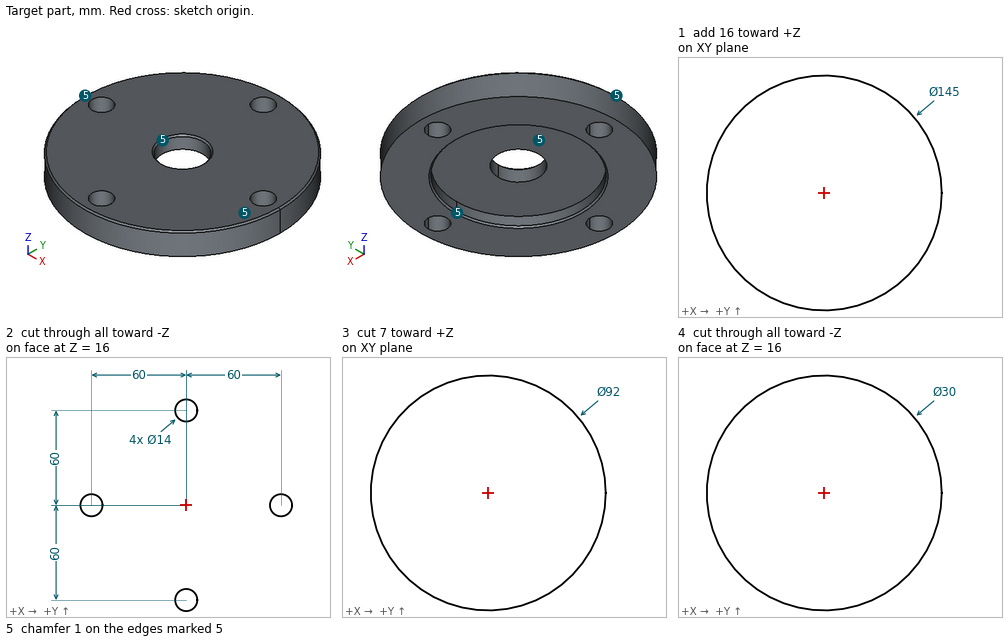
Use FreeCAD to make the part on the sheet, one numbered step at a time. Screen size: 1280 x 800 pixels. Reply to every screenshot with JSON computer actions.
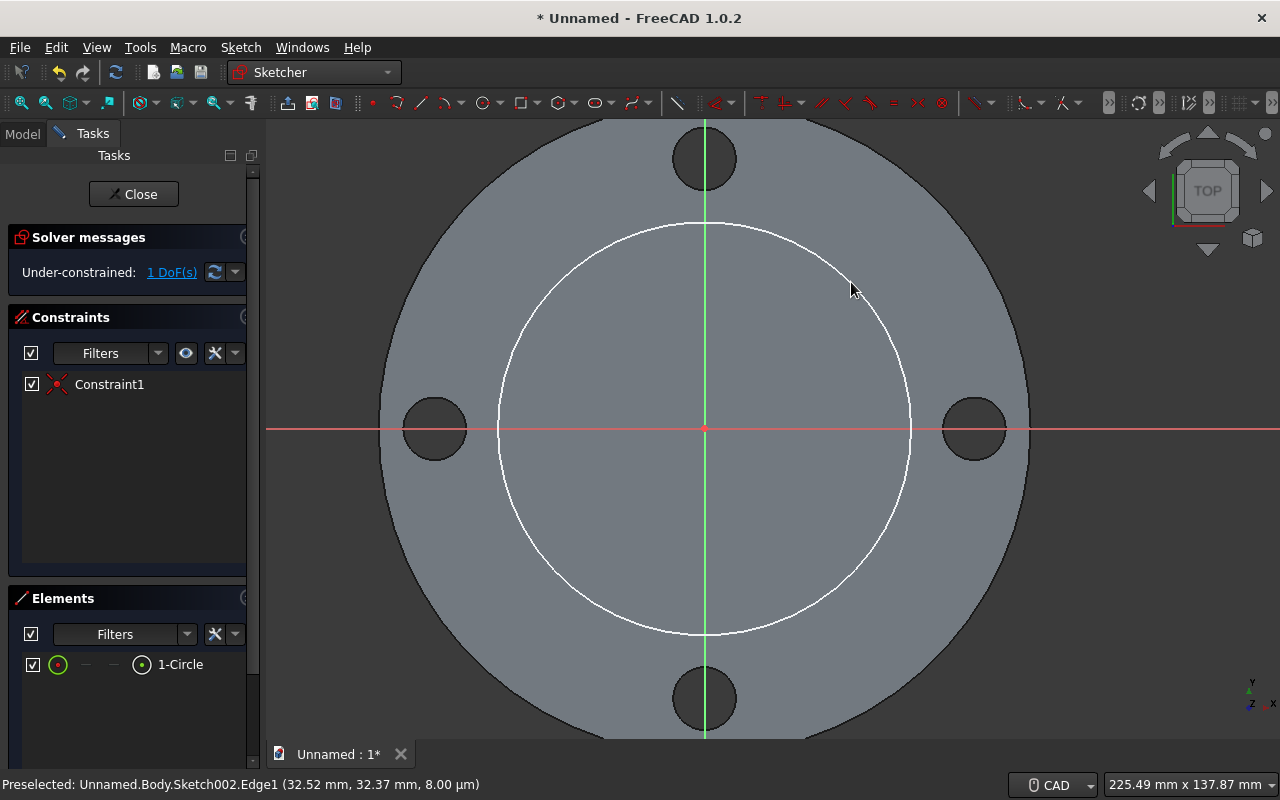
{"action": "left_click", "coordinate": [716, 104]}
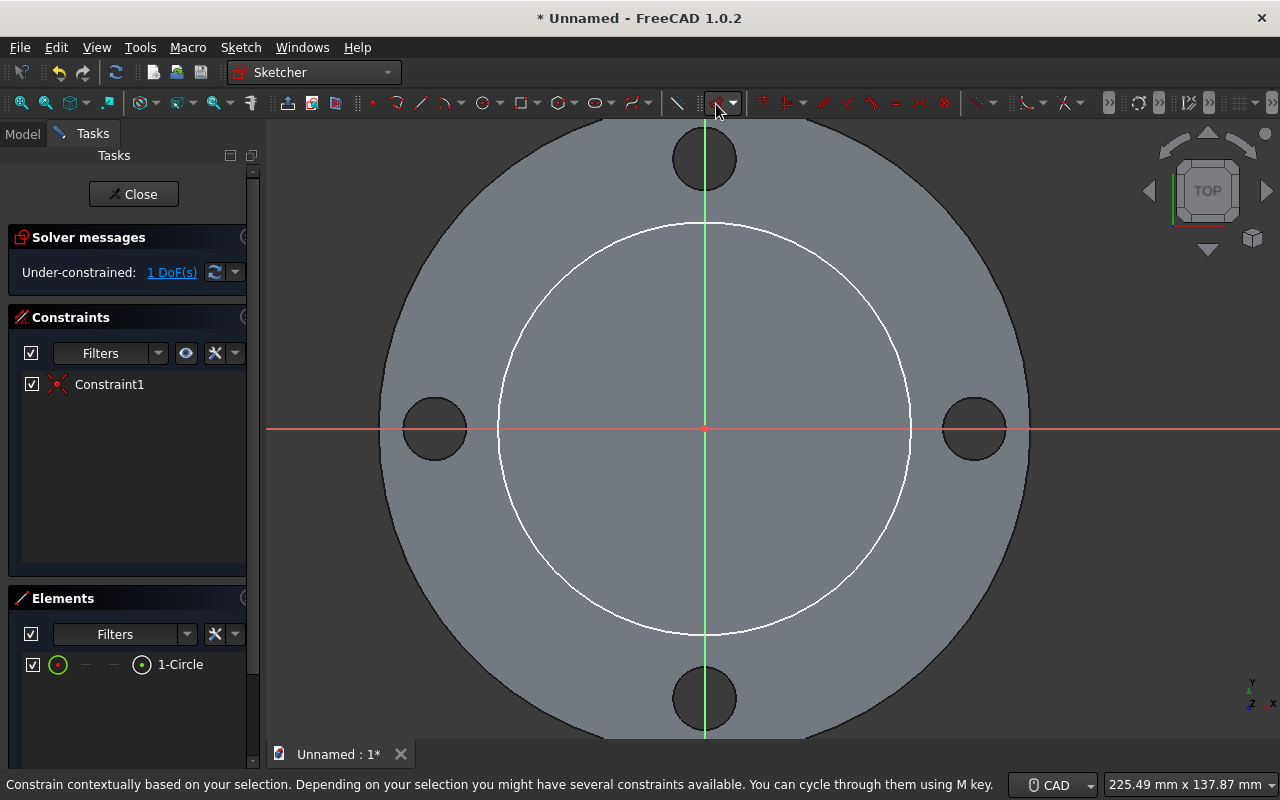
{"action": "left_click", "coordinate": [850, 282]}
{"action": "left_click", "coordinate": [873, 259]}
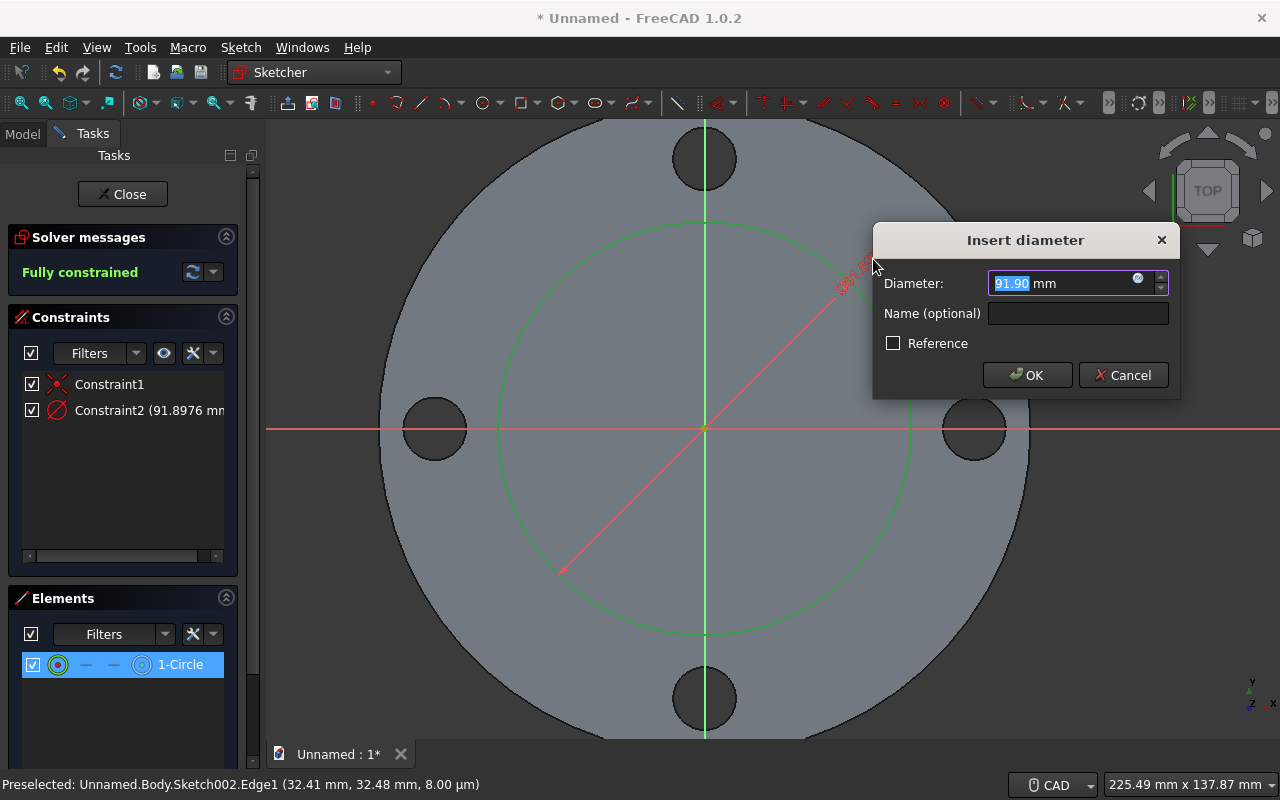
{"action": "type", "text": "92"}
{"action": "key", "text": "Return"}
{"action": "key", "text": "Escape"}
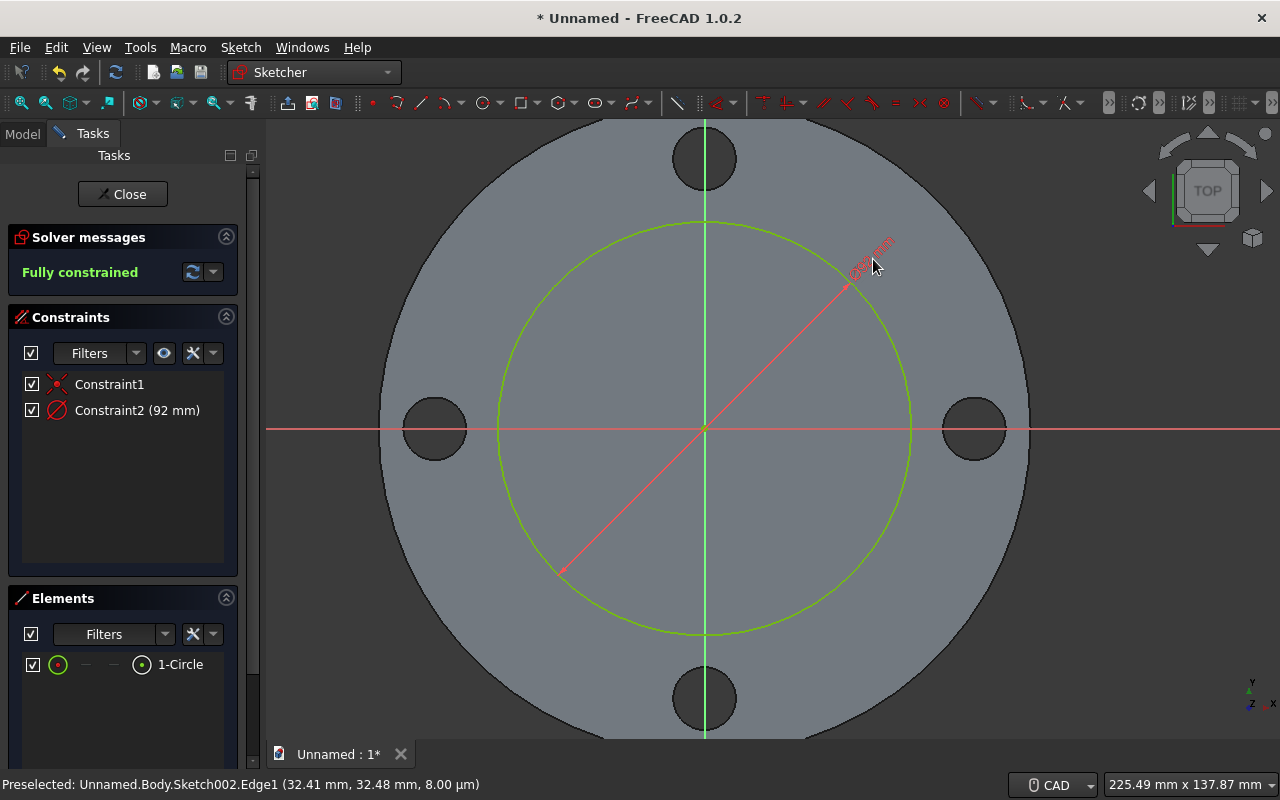
{"action": "left_click", "coordinate": [123, 194]}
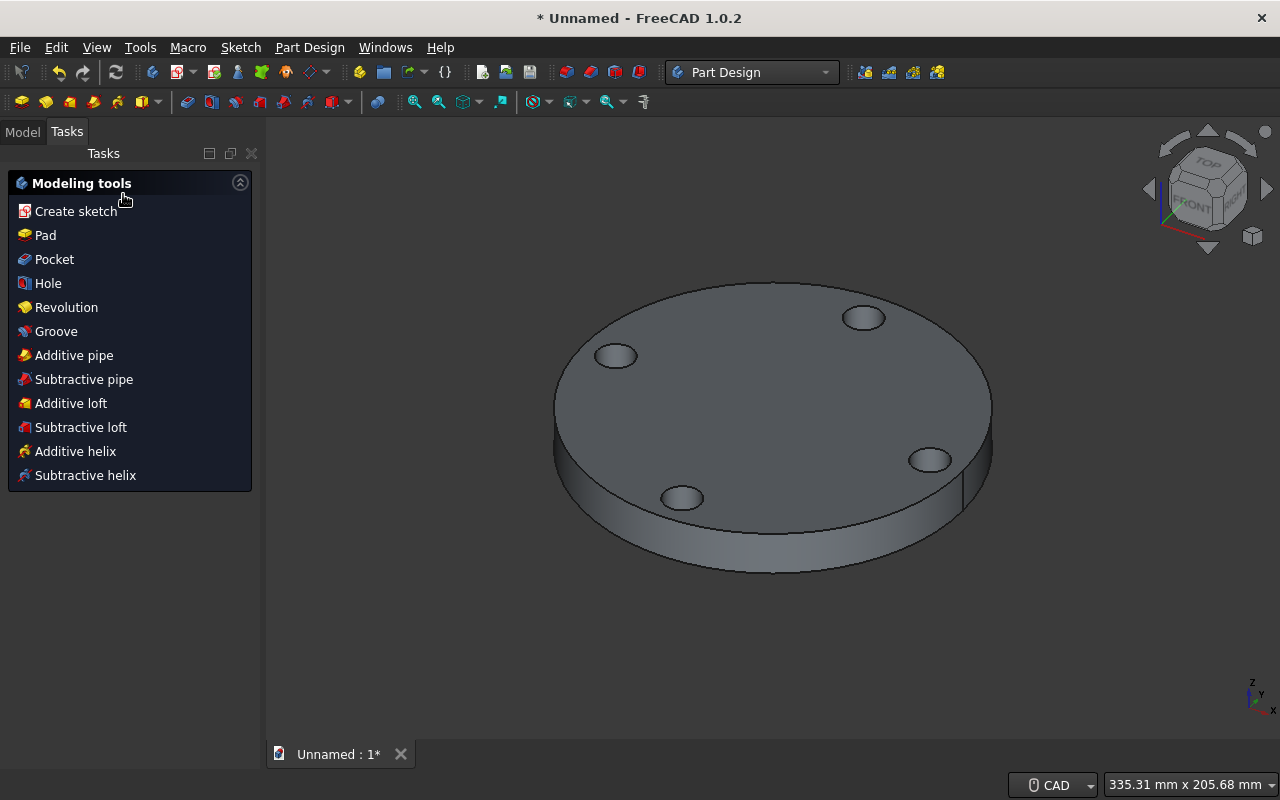
{"action": "left_click", "coordinate": [188, 102]}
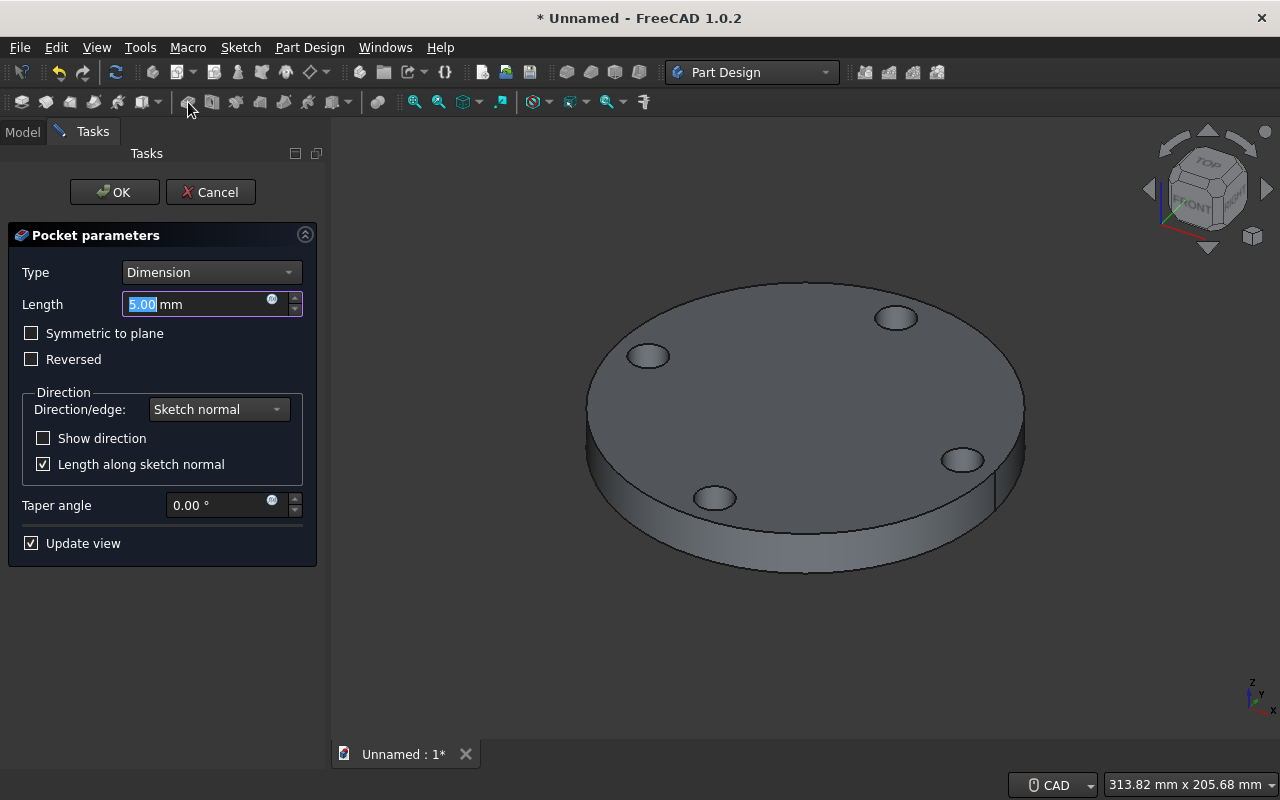
{"action": "type", "text": "7"}
{"action": "key", "text": "Tab"}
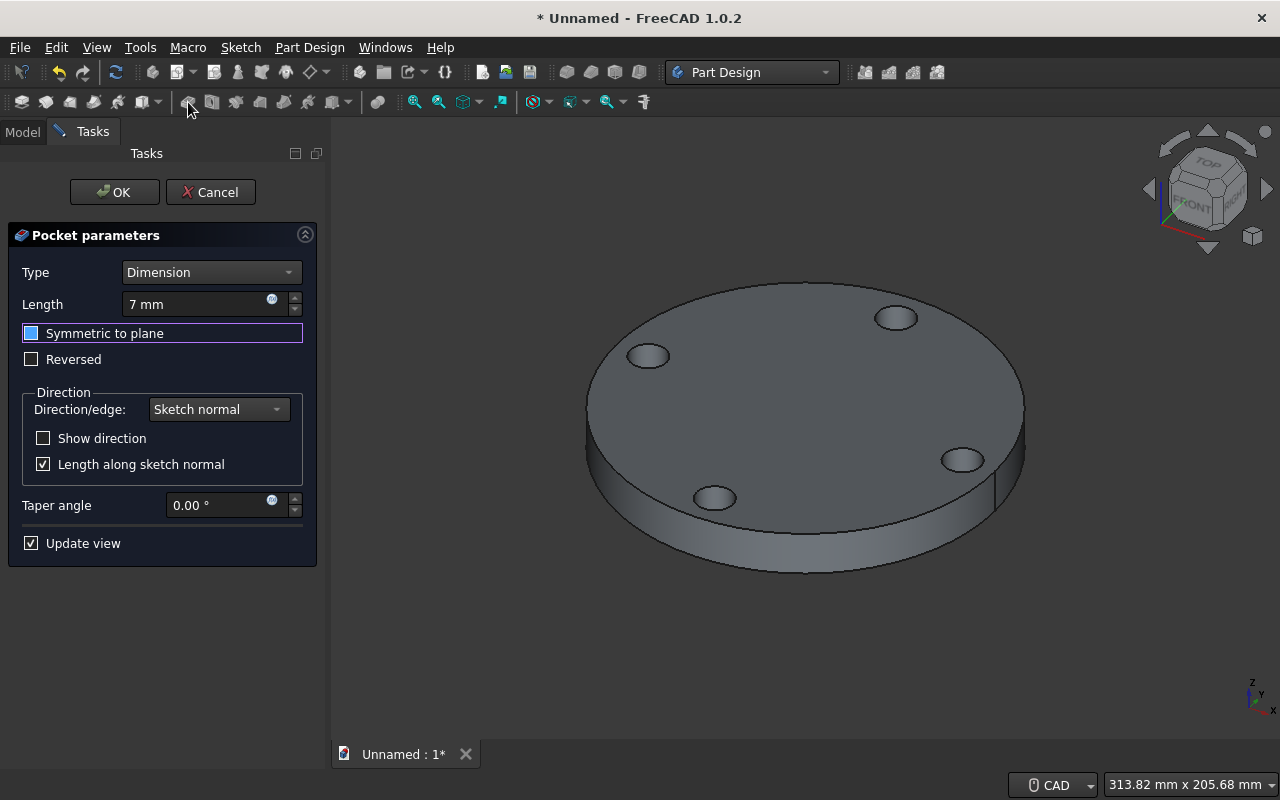
{"action": "left_click", "coordinate": [30, 359]}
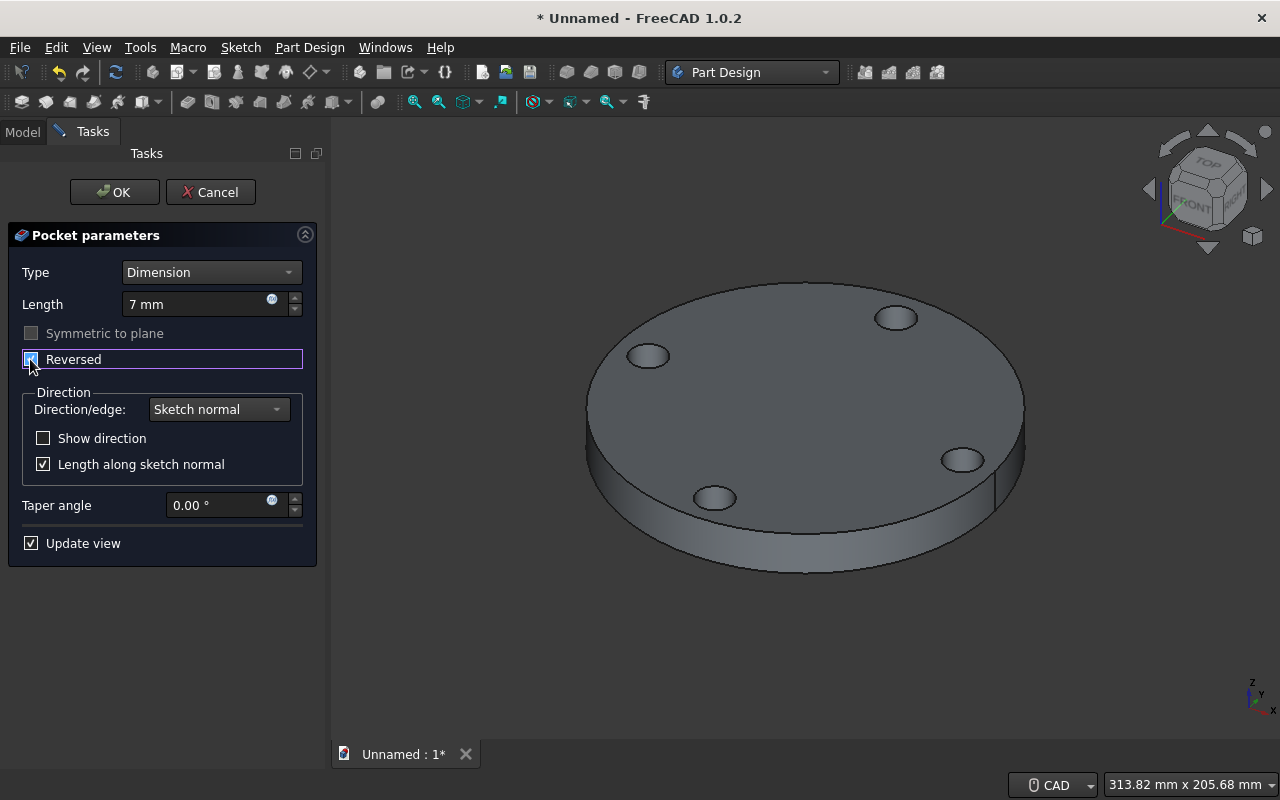
{"action": "left_click", "coordinate": [115, 192]}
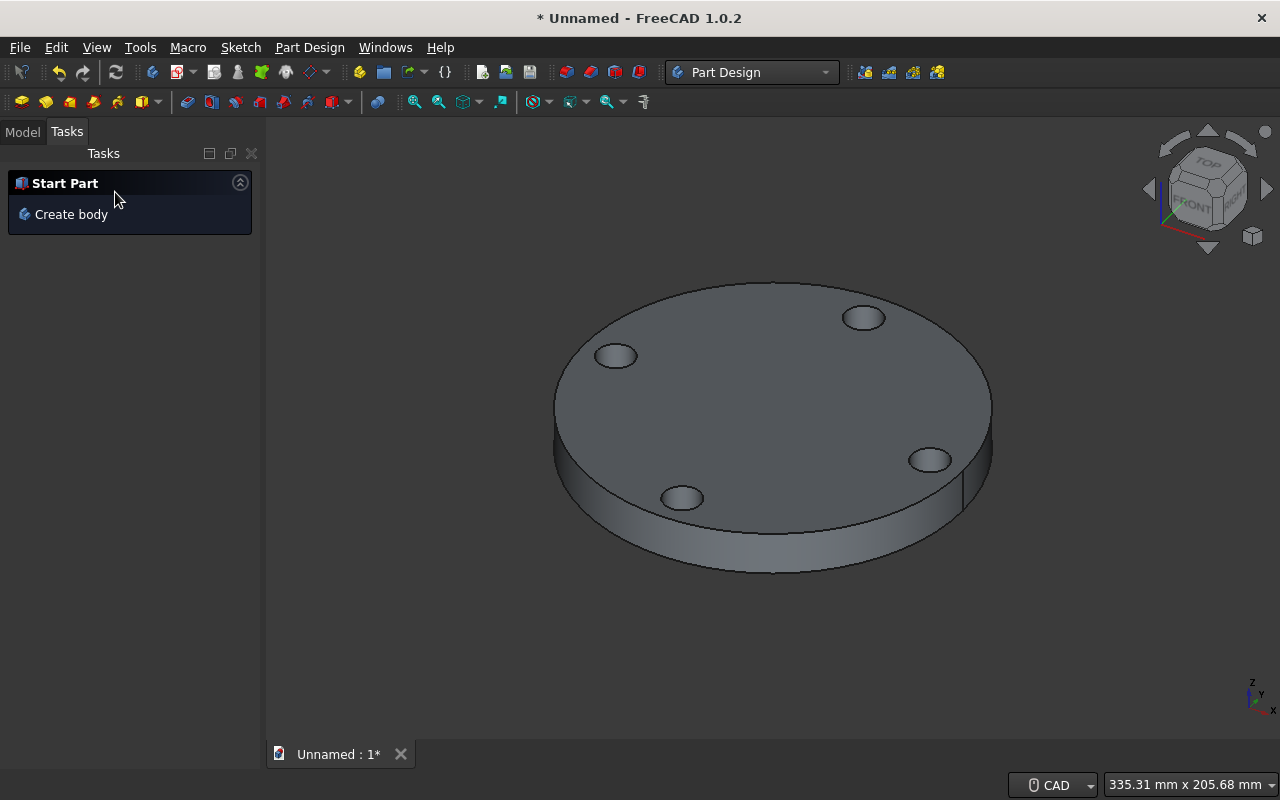
{"action": "left_click", "coordinate": [773, 407]}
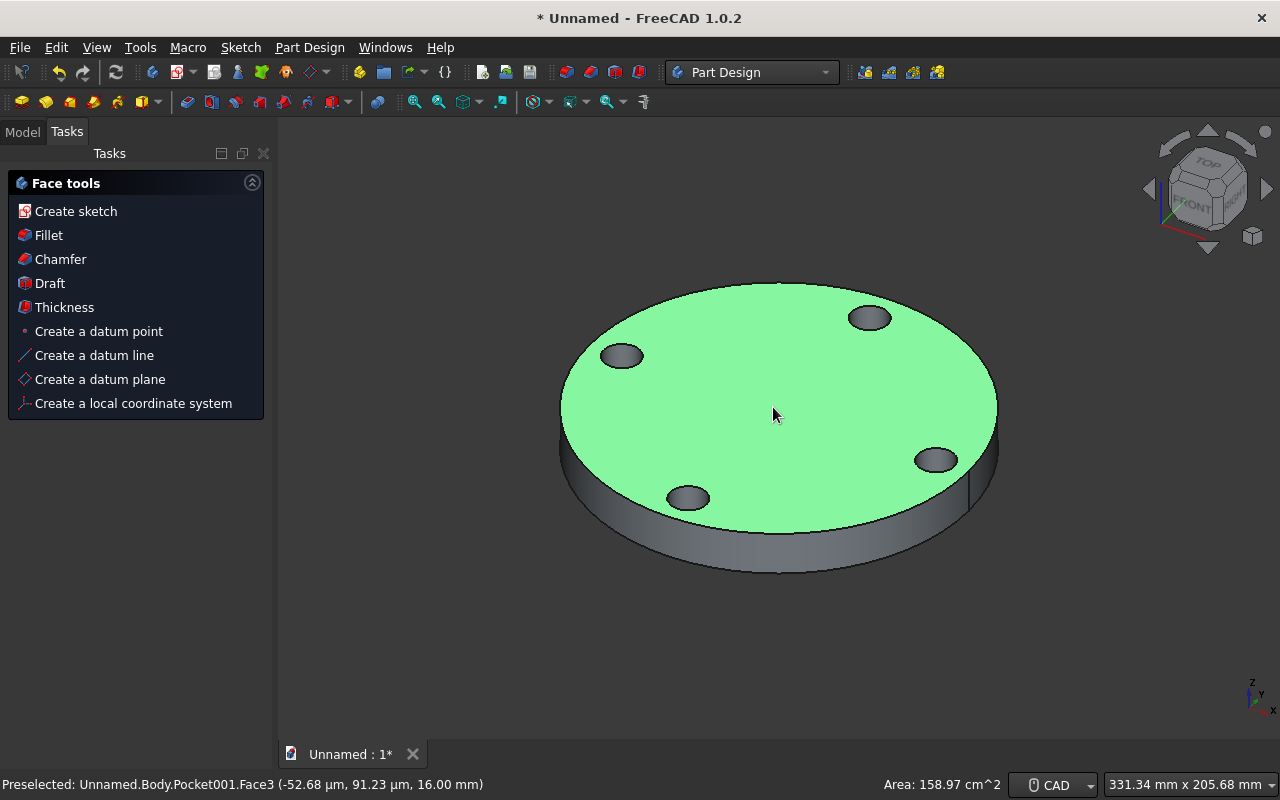
{"action": "left_click", "coordinate": [178, 72]}